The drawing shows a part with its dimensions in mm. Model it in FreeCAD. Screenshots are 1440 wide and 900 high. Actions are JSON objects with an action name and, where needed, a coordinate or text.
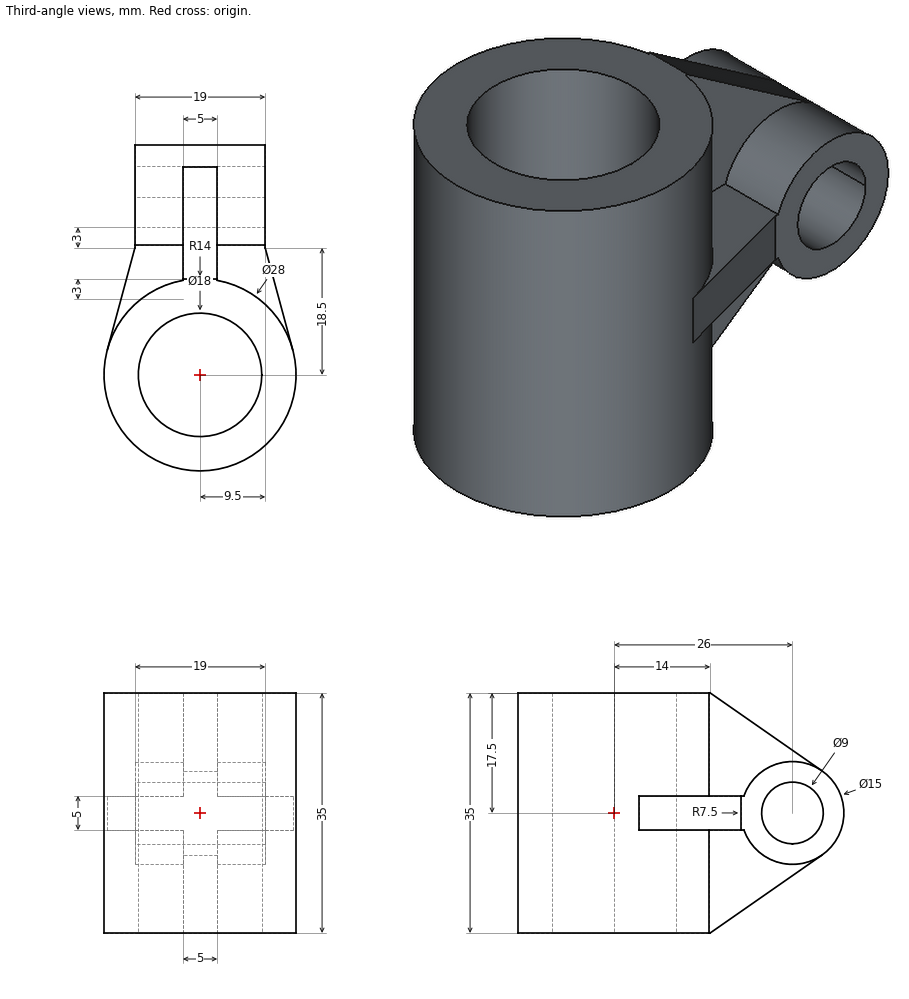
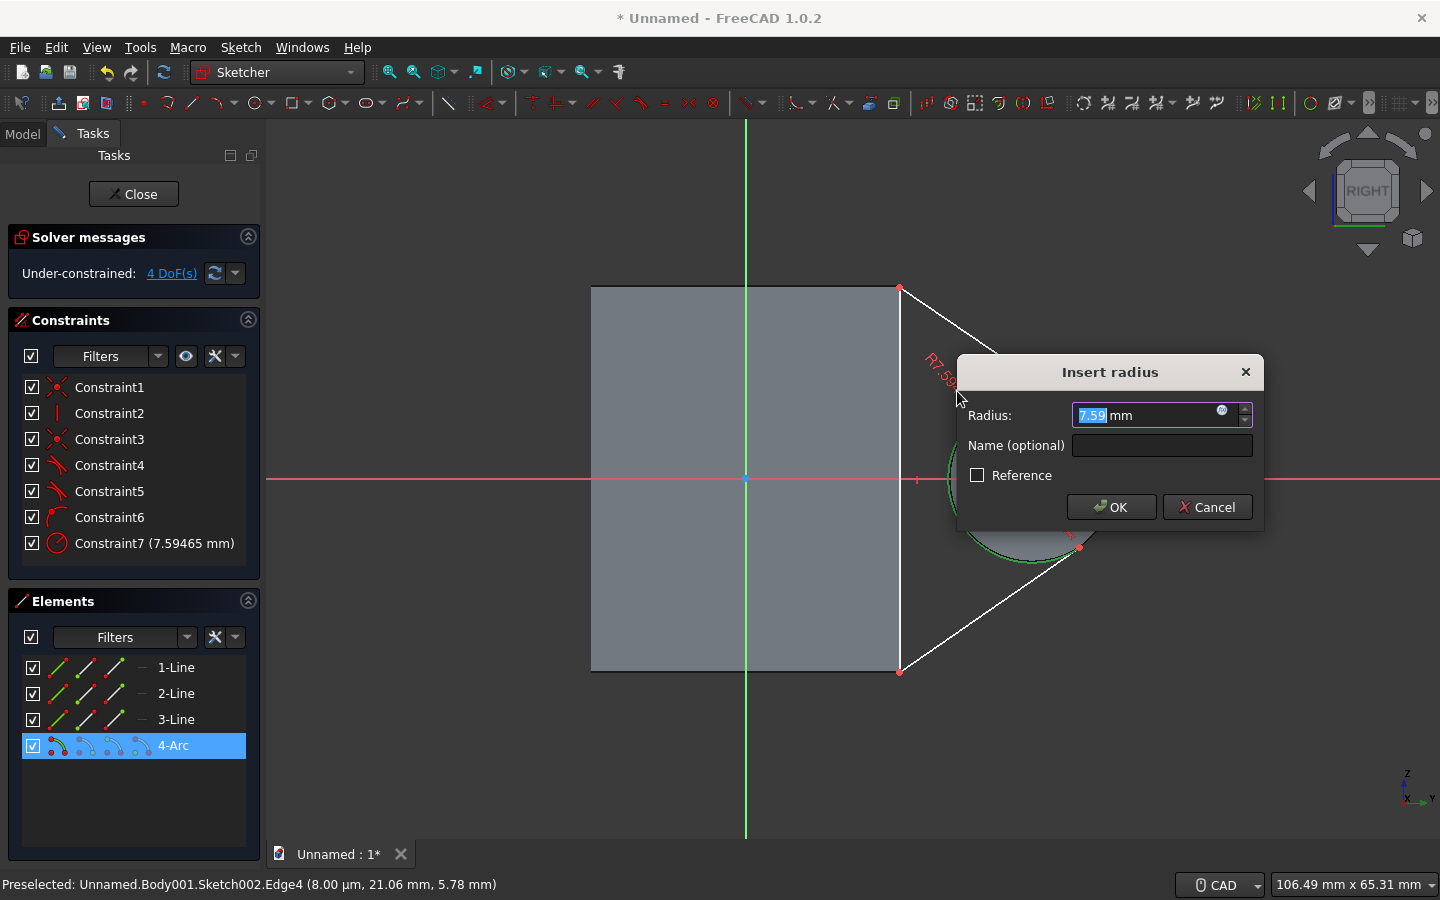
{"action": "type", "text": "7.5"}
{"action": "key", "text": "Return"}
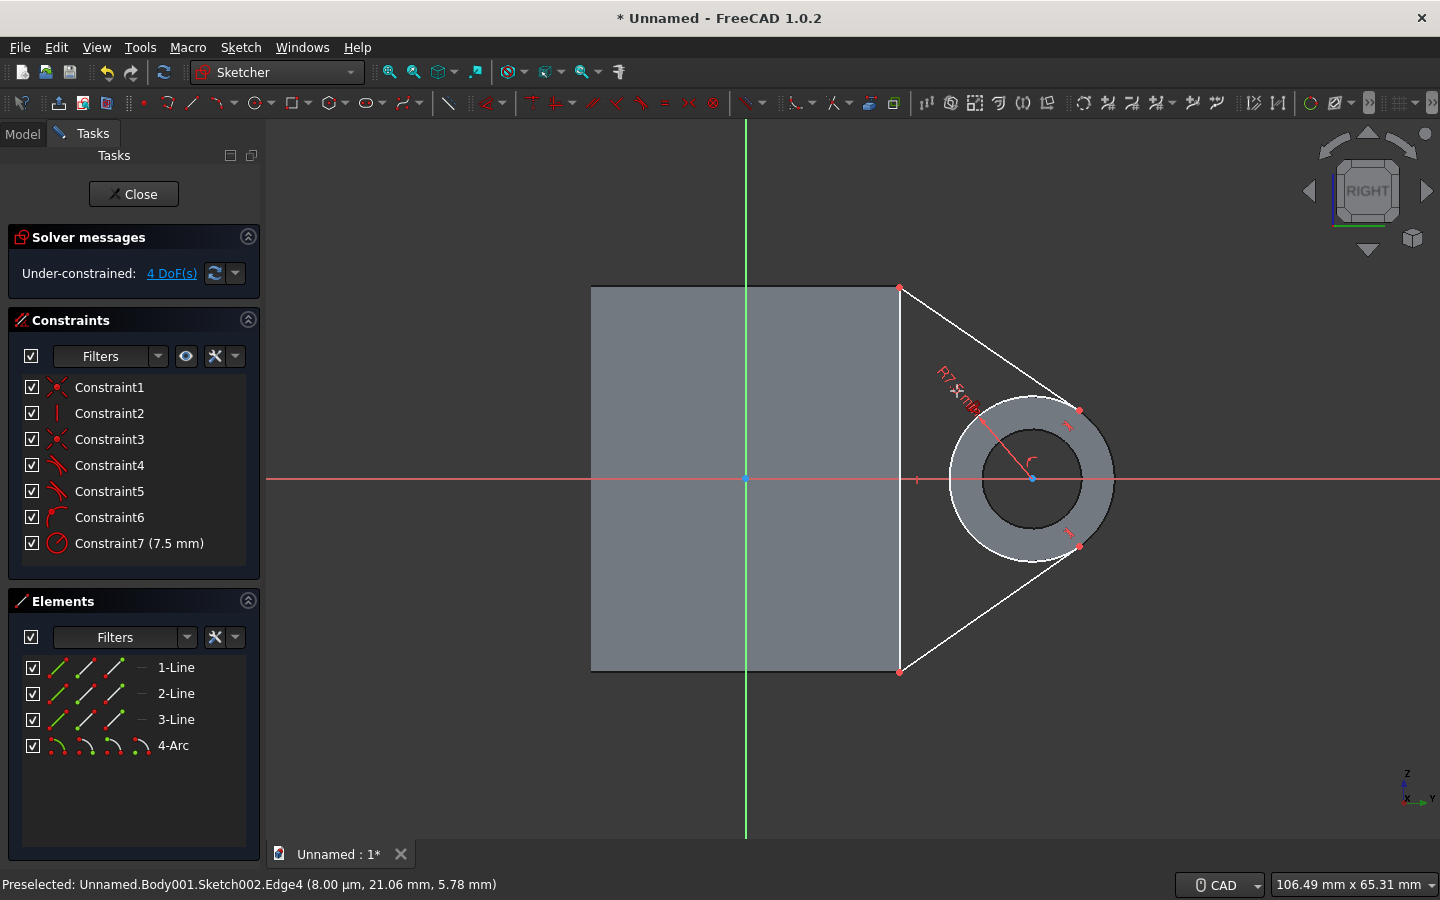
{"action": "left_click", "coordinate": [900, 403]}
{"action": "left_click", "coordinate": [866, 391]}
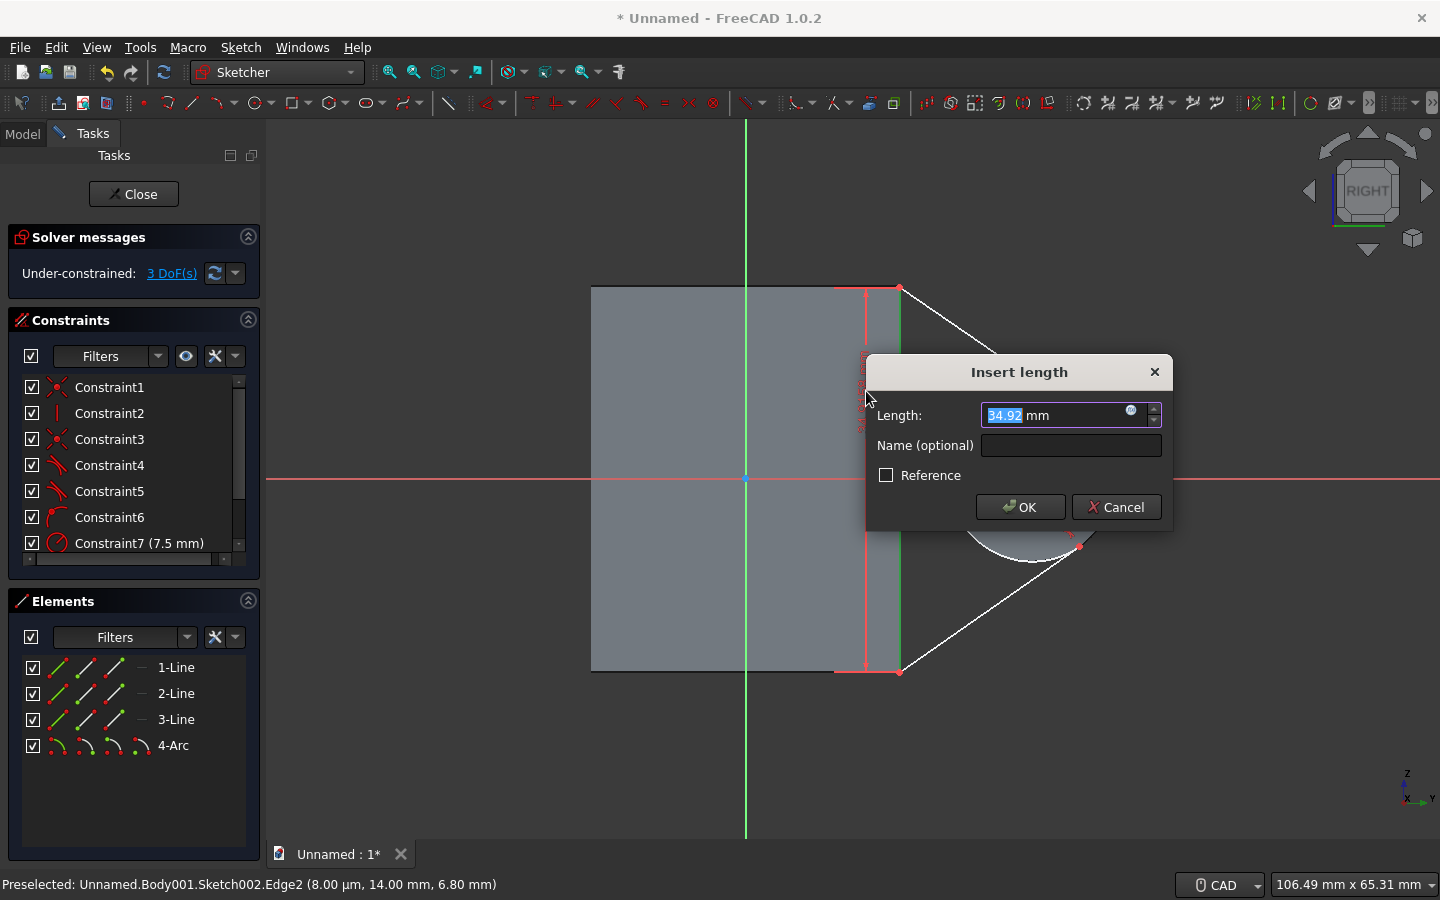
{"action": "type", "text": "35"}
{"action": "key", "text": "Return"}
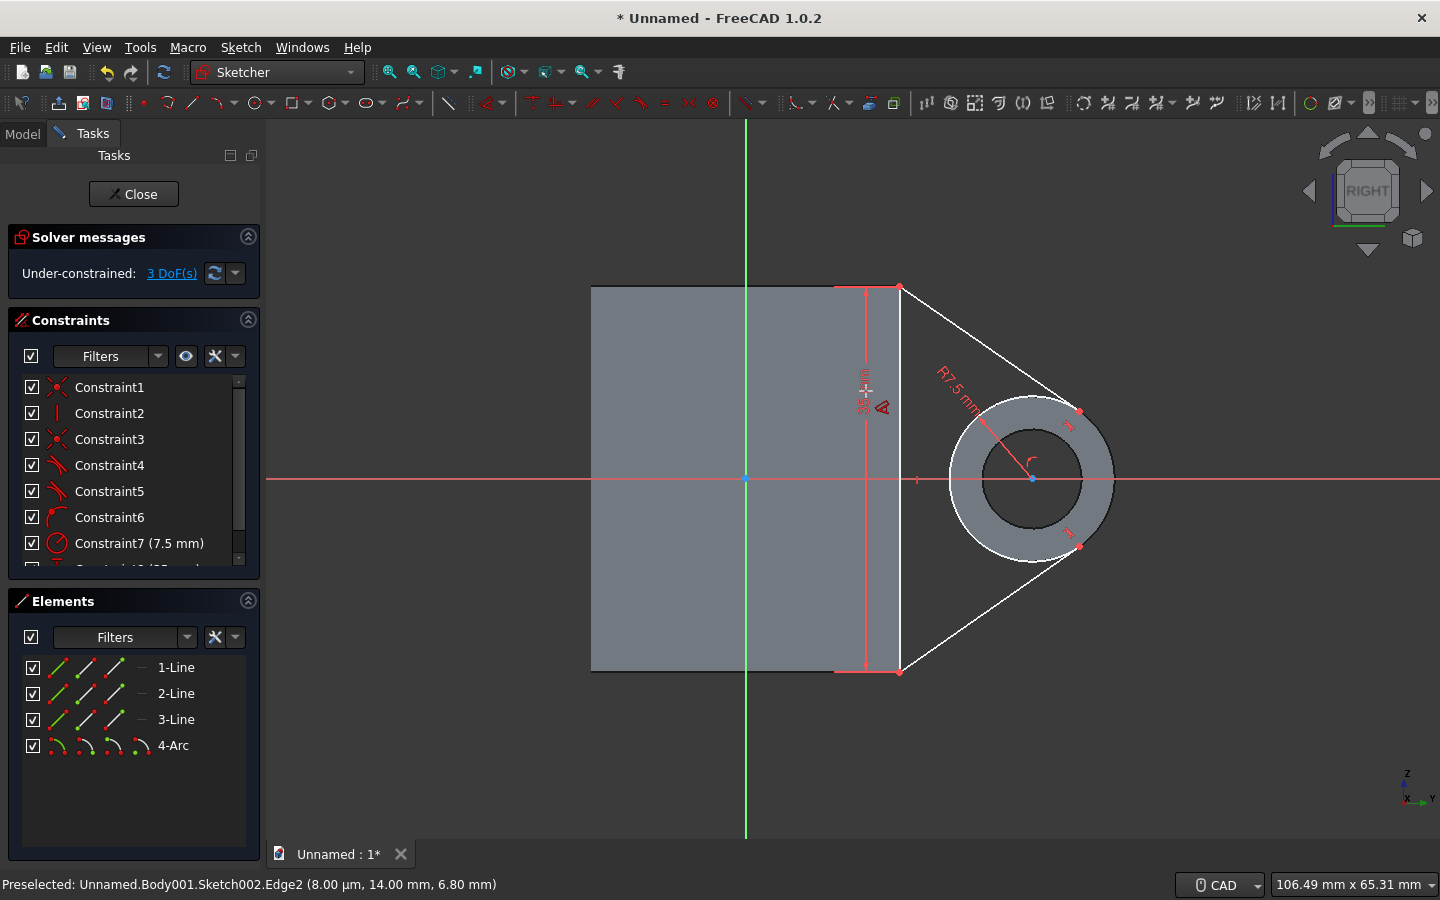
{"action": "left_click", "coordinate": [900, 287]}
{"action": "left_click", "coordinate": [823, 253]}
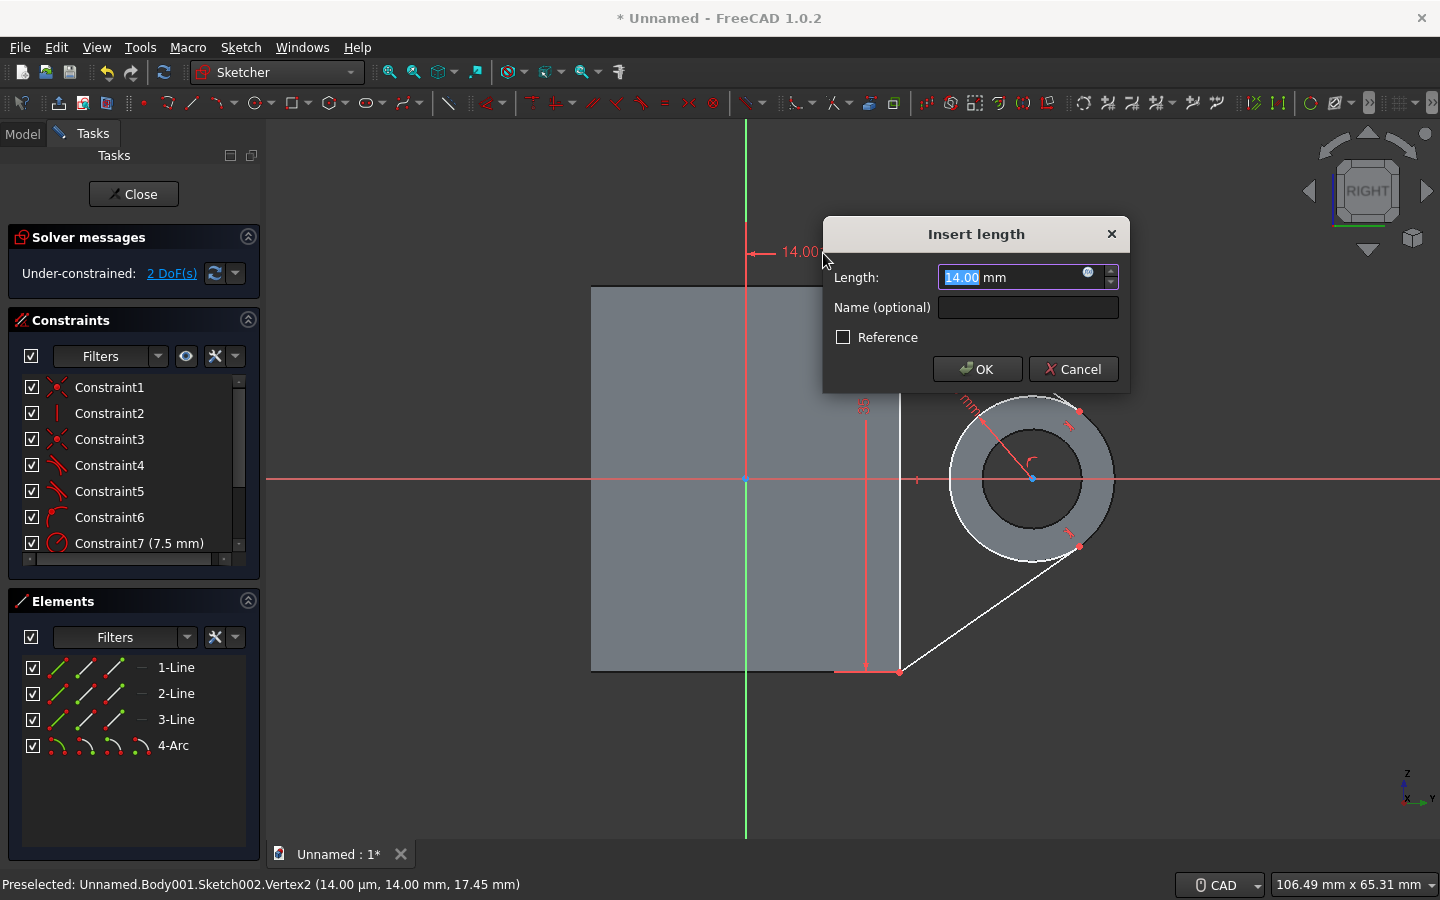
{"action": "type", "text": "14"}
{"action": "key", "text": "Return"}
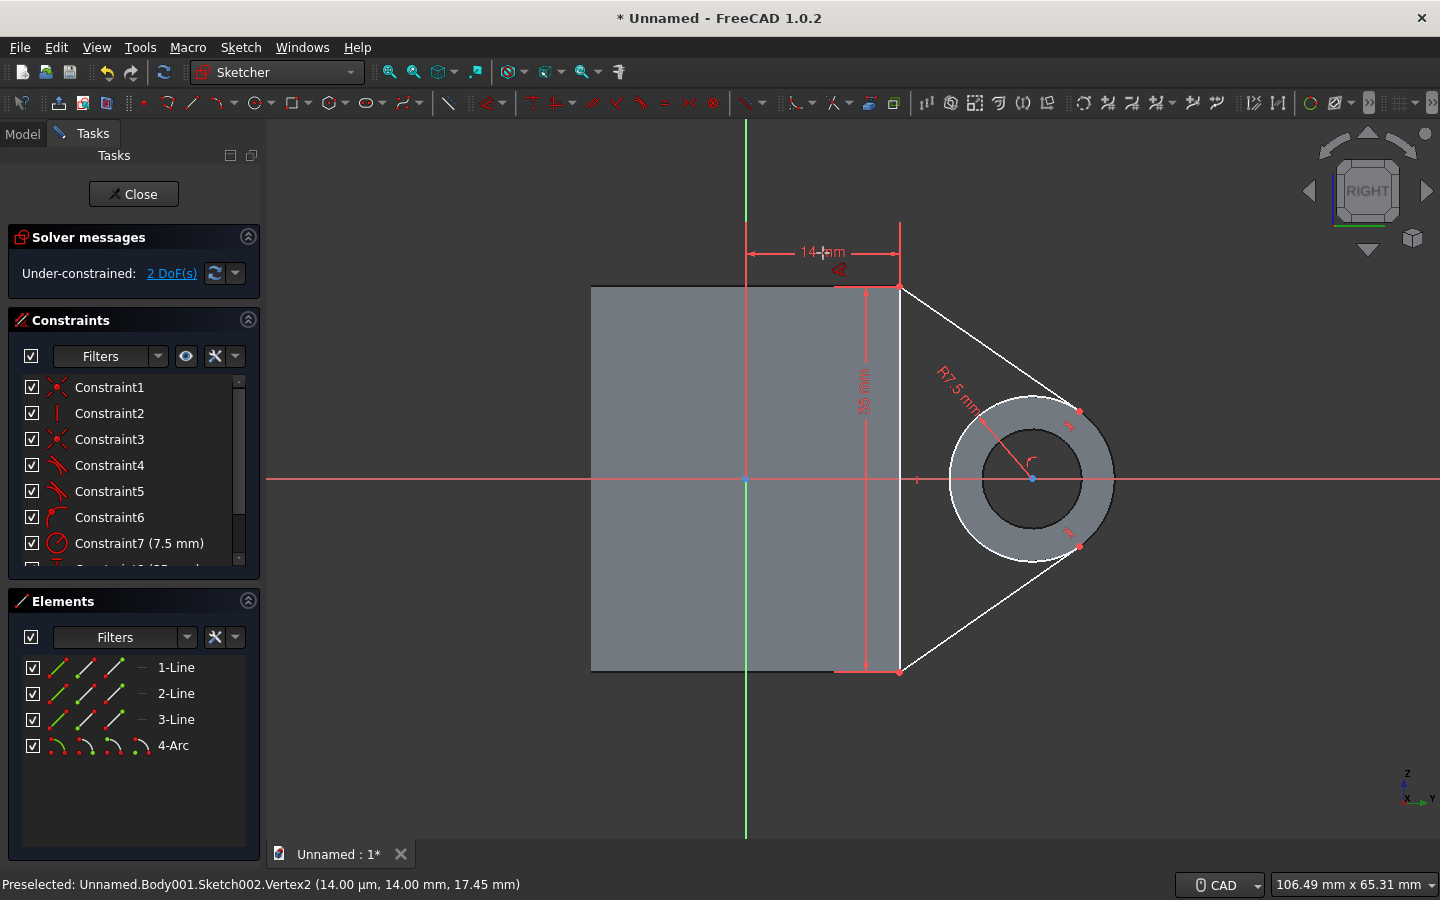
{"action": "left_click", "coordinate": [1032, 479]}
{"action": "left_click", "coordinate": [823, 513]}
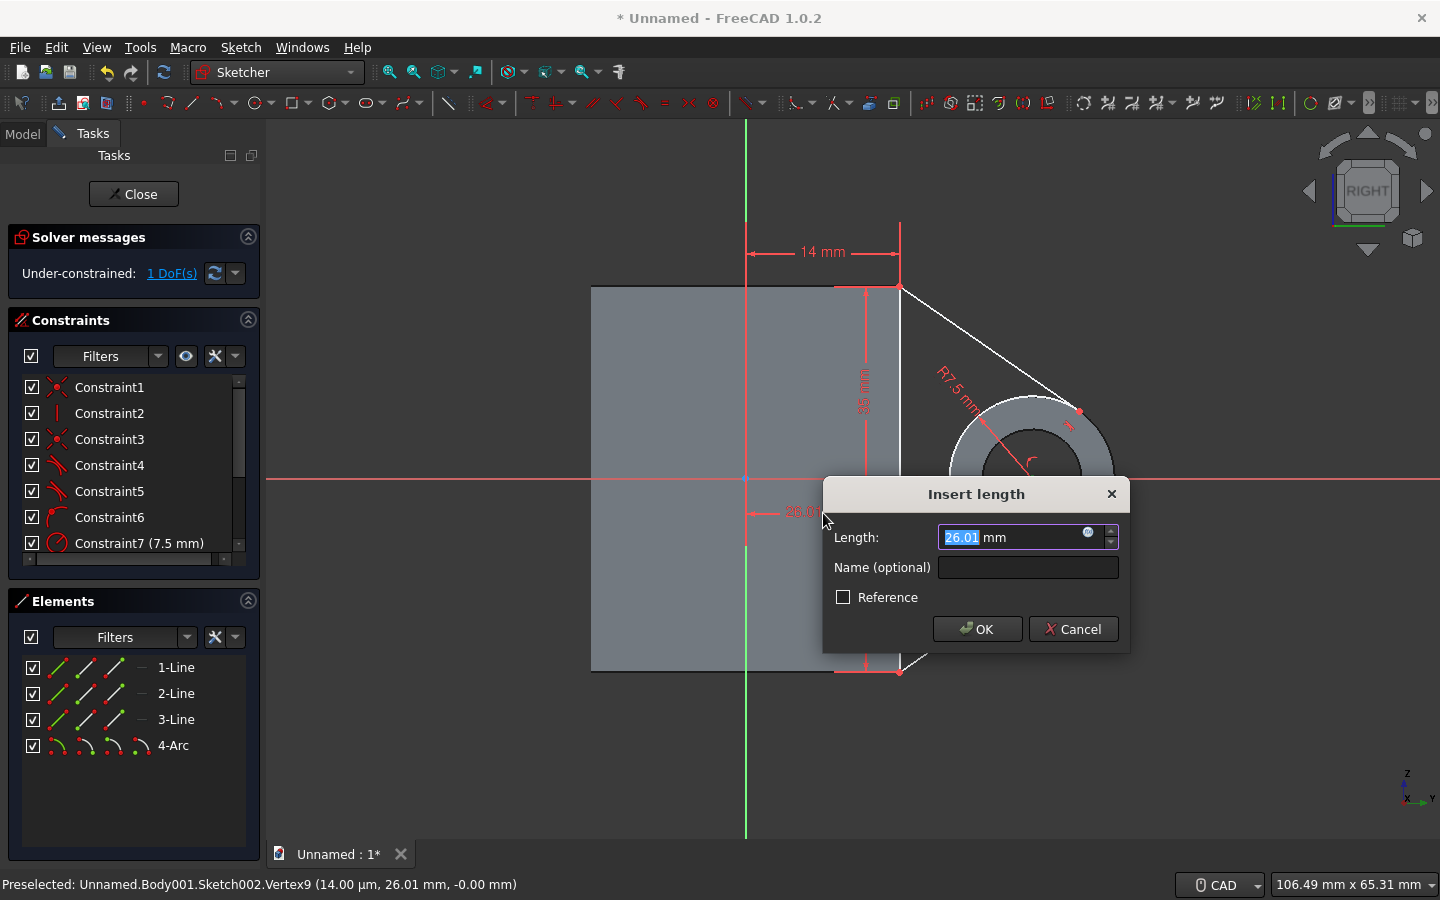
{"action": "type", "text": "26"}
{"action": "key", "text": "Return"}